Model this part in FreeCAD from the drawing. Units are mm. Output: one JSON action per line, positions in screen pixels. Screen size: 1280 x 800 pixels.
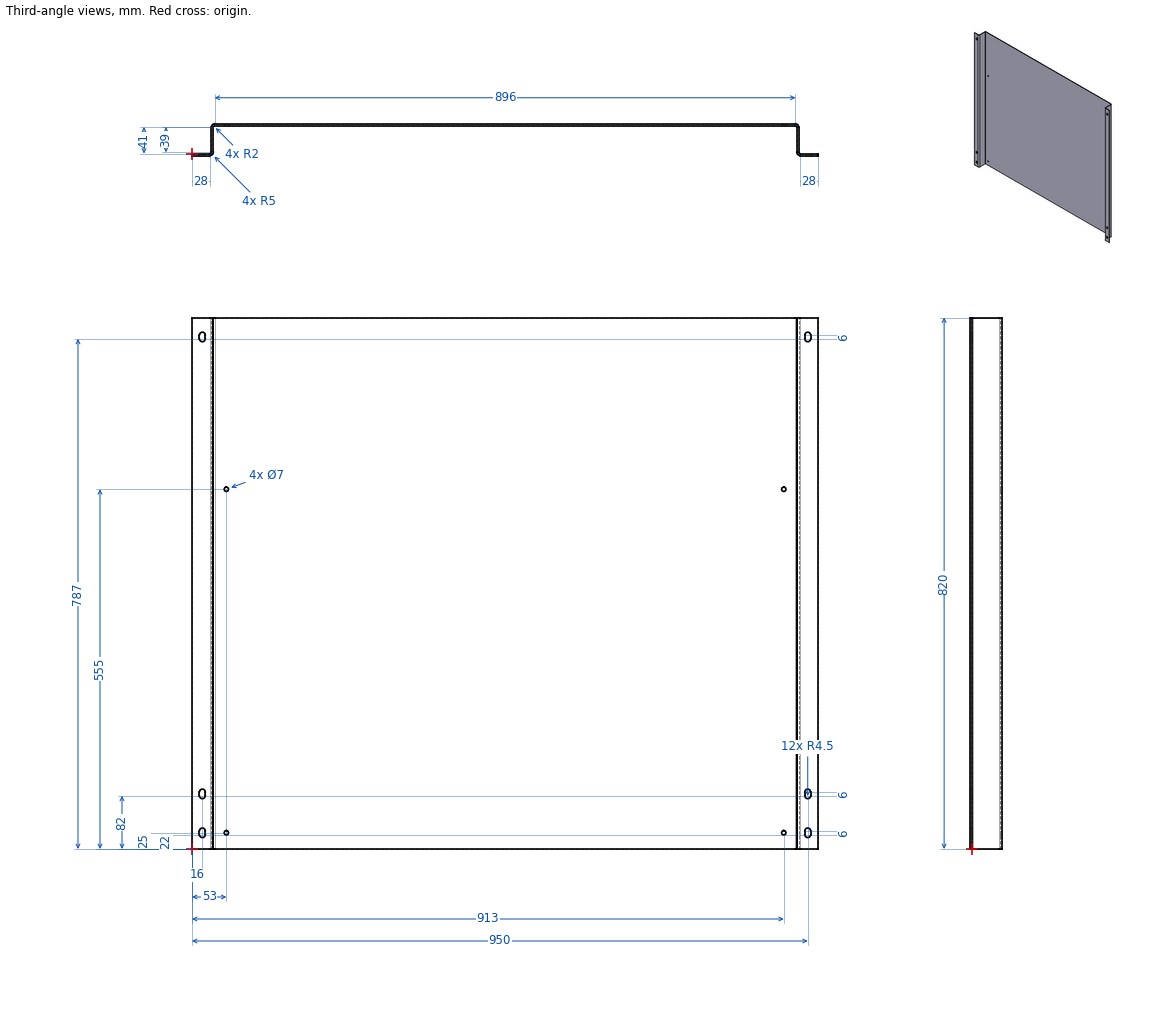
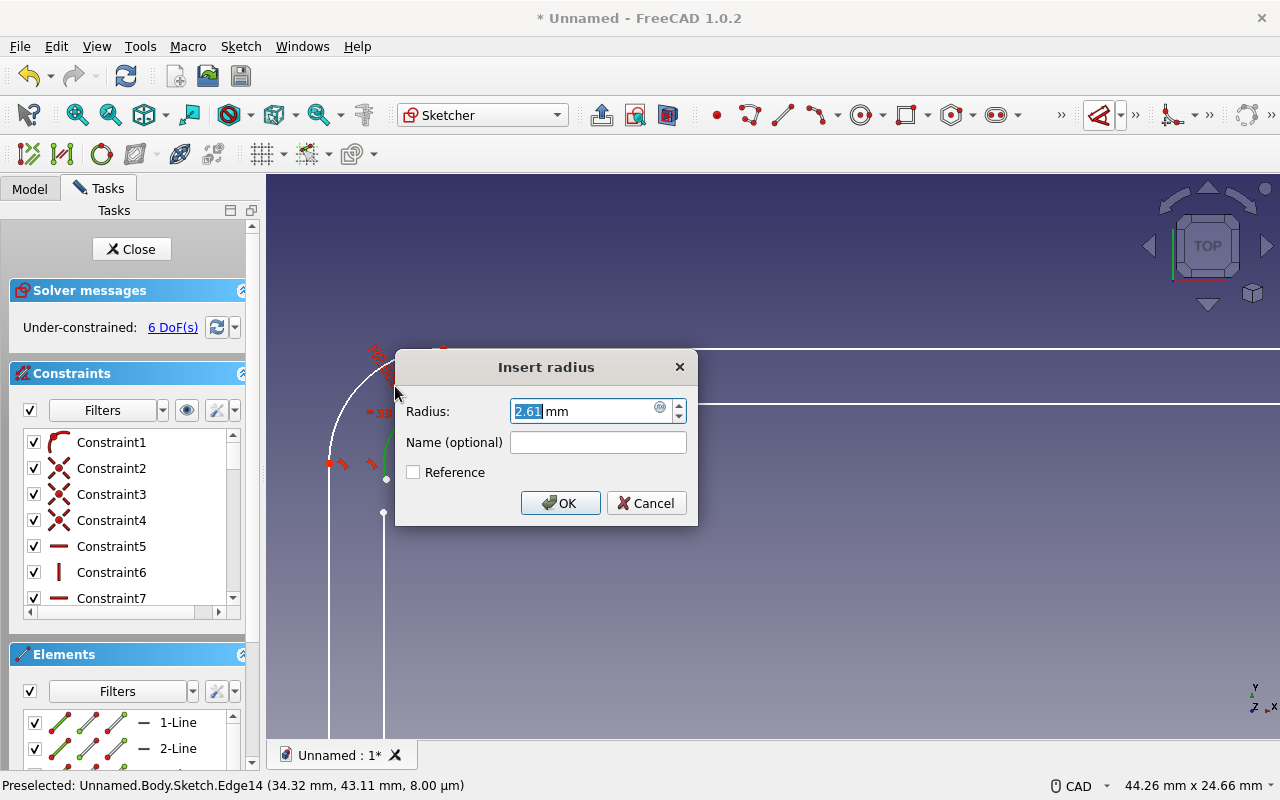
{"action": "type", "text": "2"}
{"action": "key", "text": "Return"}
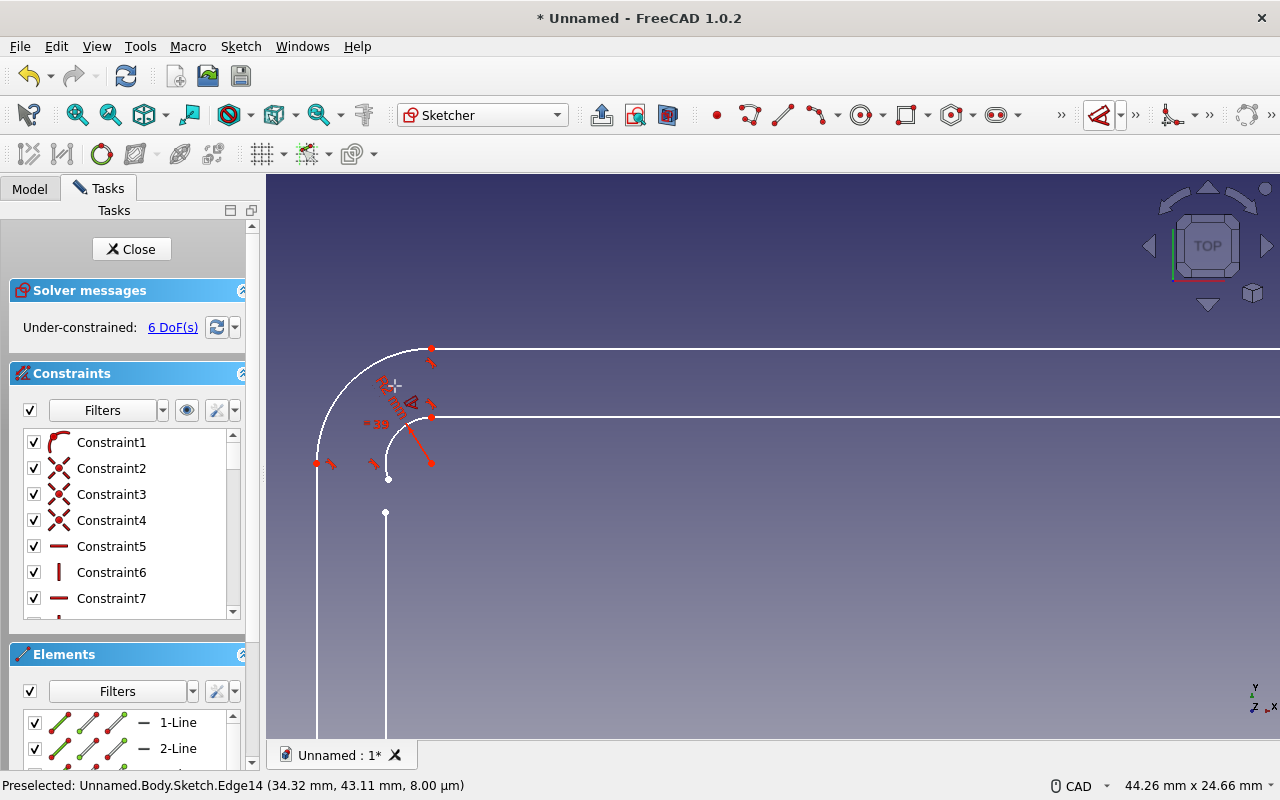
{"action": "scroll", "coordinate": [360, 441], "scroll_direction": "down", "scroll_amount": 17}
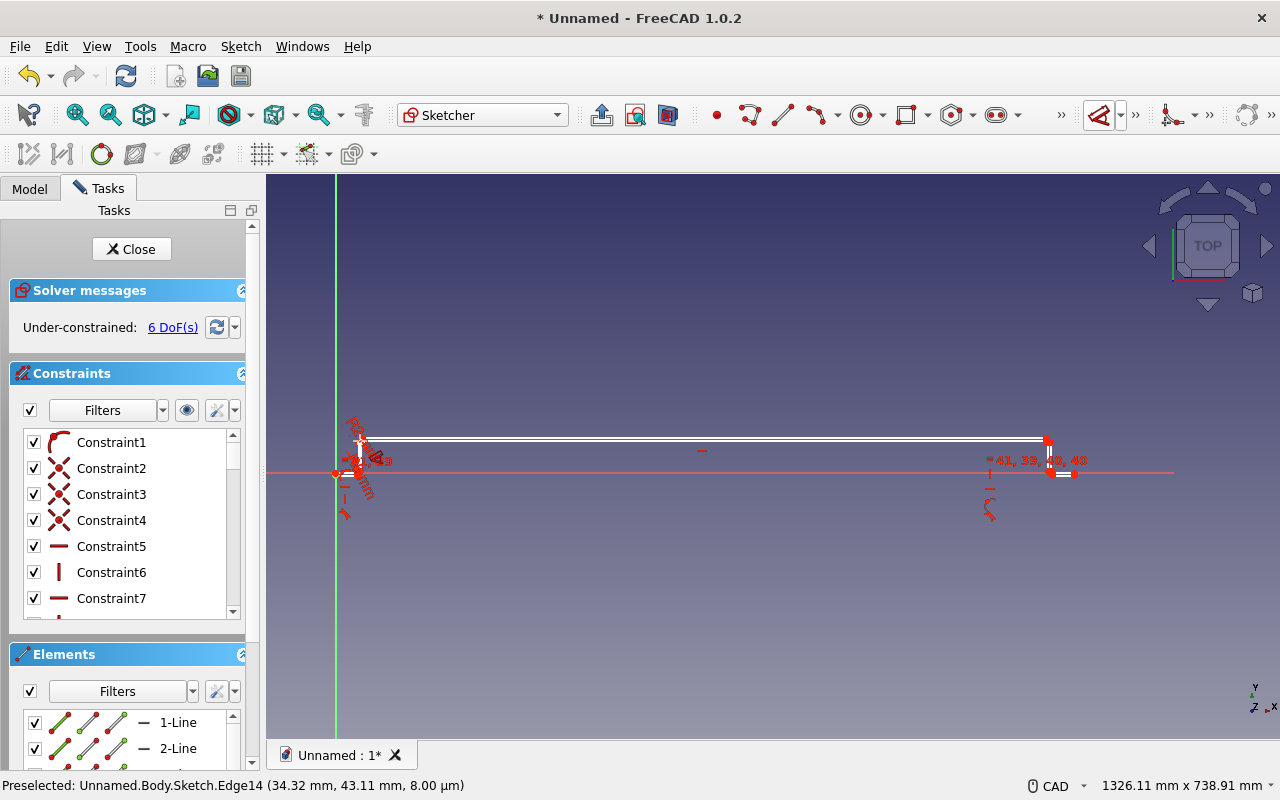
{"action": "scroll", "coordinate": [351, 473], "scroll_direction": "up", "scroll_amount": 9}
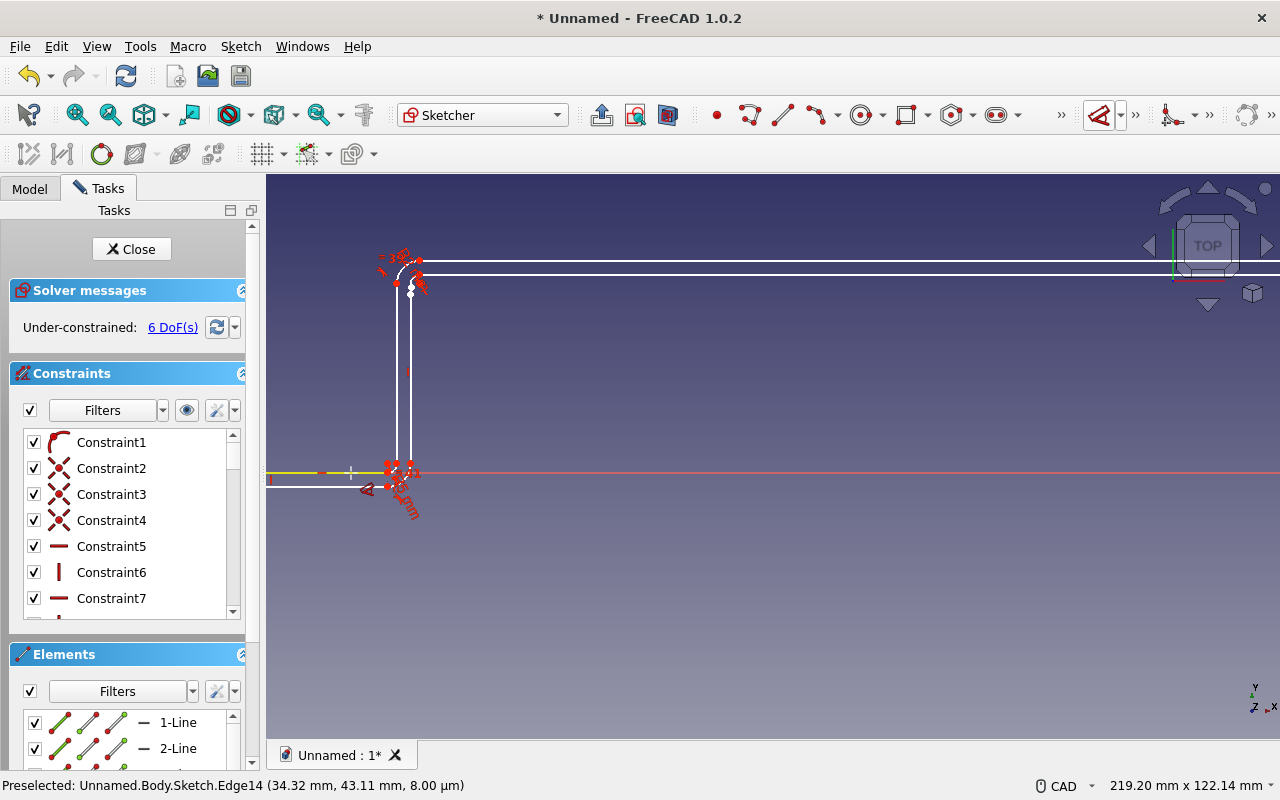
{"action": "left_click", "coordinate": [349, 473]}
{"action": "left_click", "coordinate": [319, 507]}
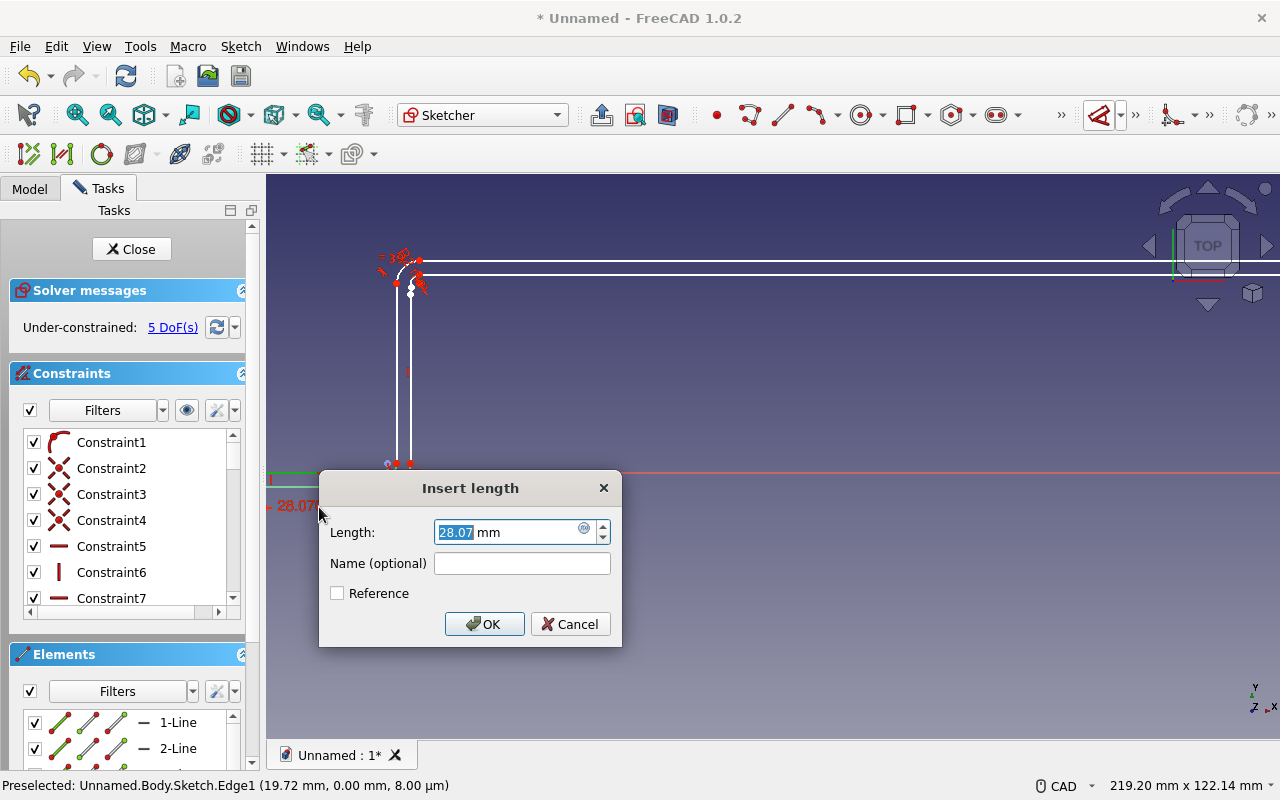
{"action": "type", "text": "28"}
{"action": "key", "text": "Return"}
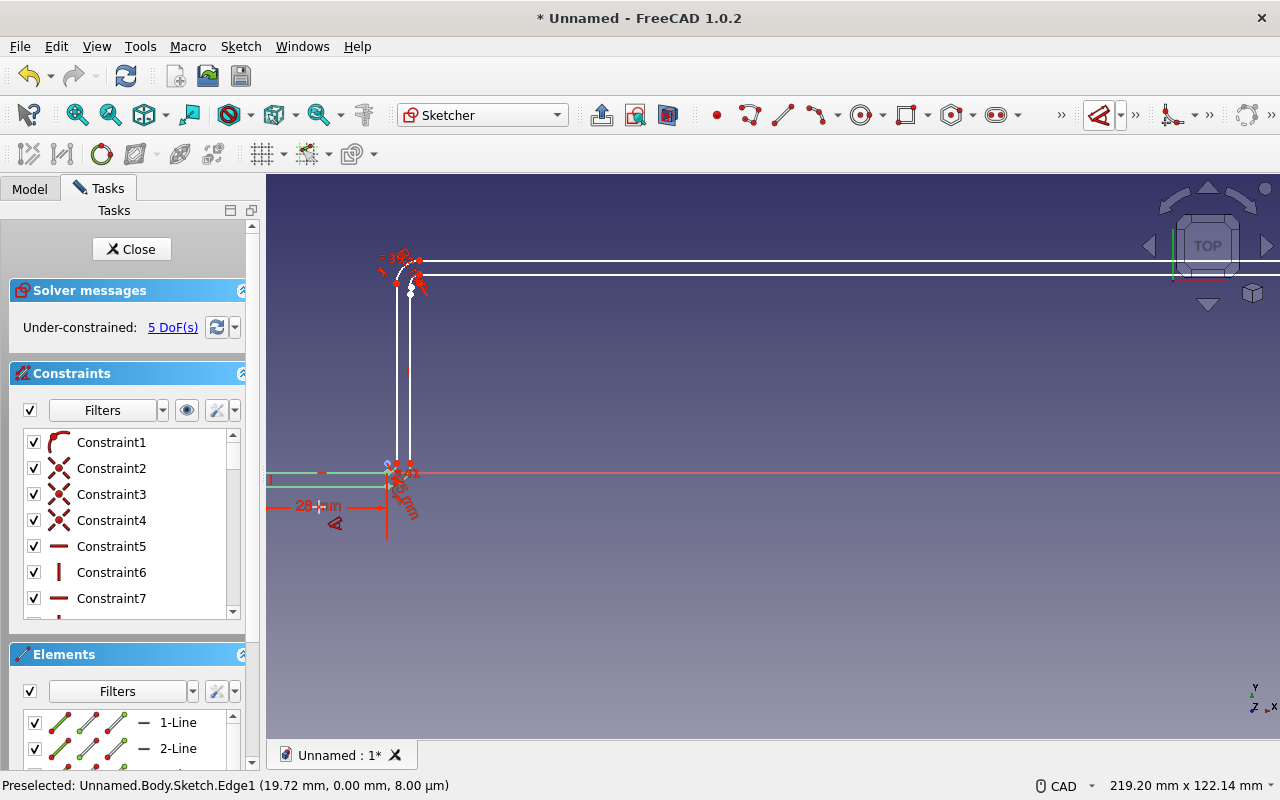
{"action": "left_click", "coordinate": [410, 413]}
{"action": "left_click", "coordinate": [376, 379]}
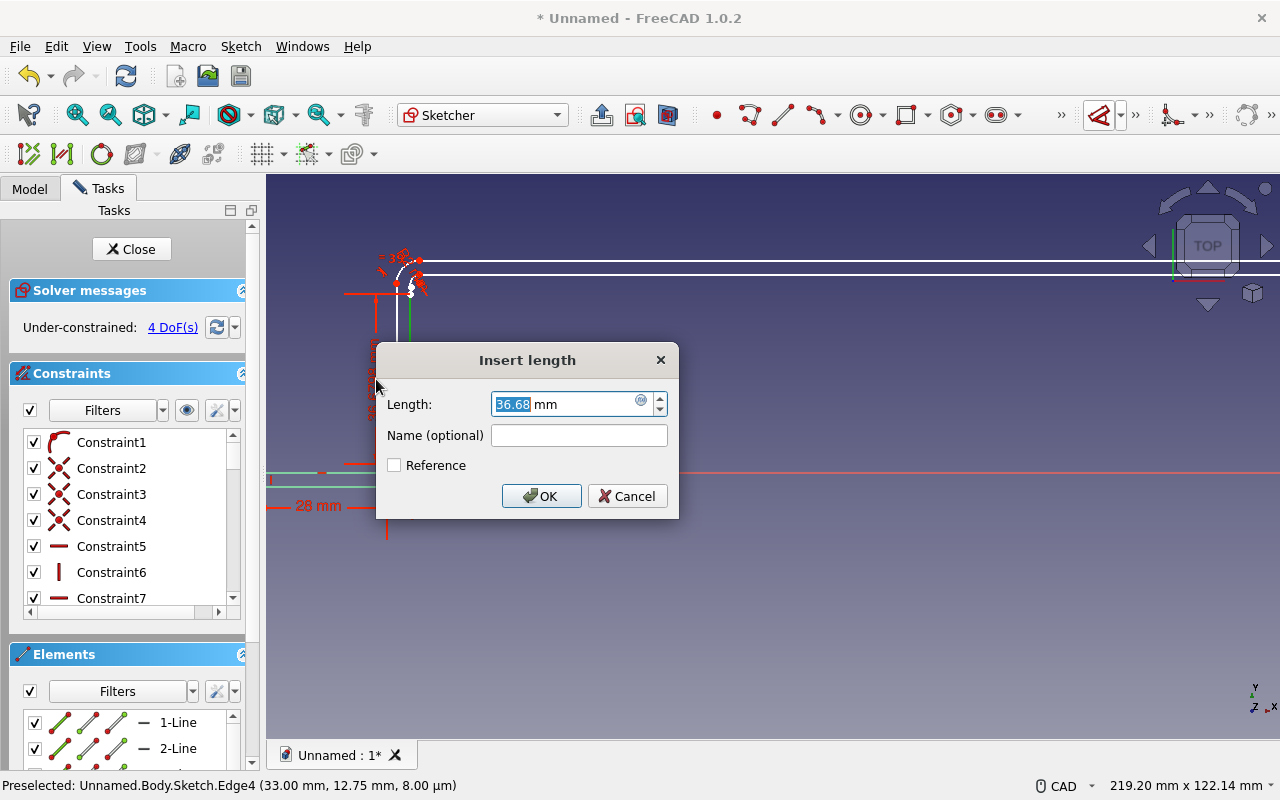
{"action": "type", "text": "39"}
{"action": "key", "text": "Return"}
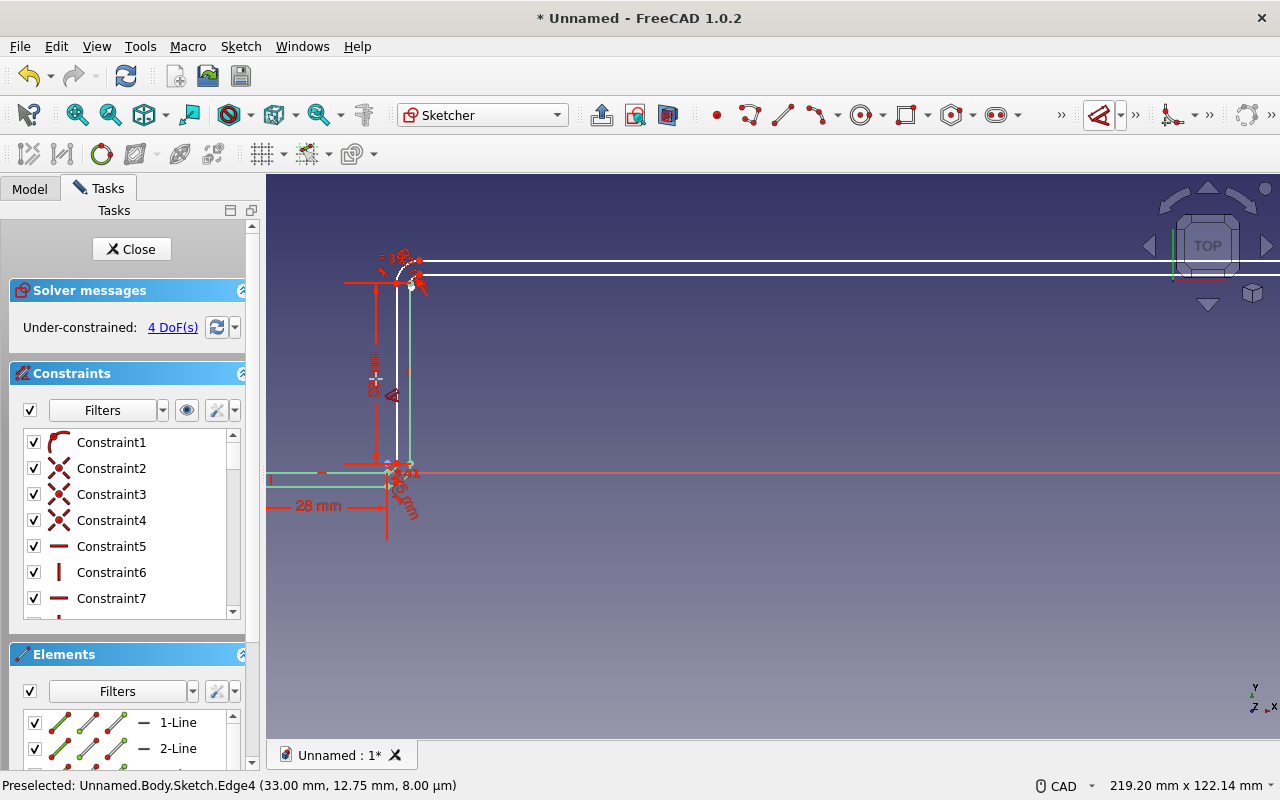
{"action": "scroll", "coordinate": [425, 469], "scroll_direction": "down", "scroll_amount": 10}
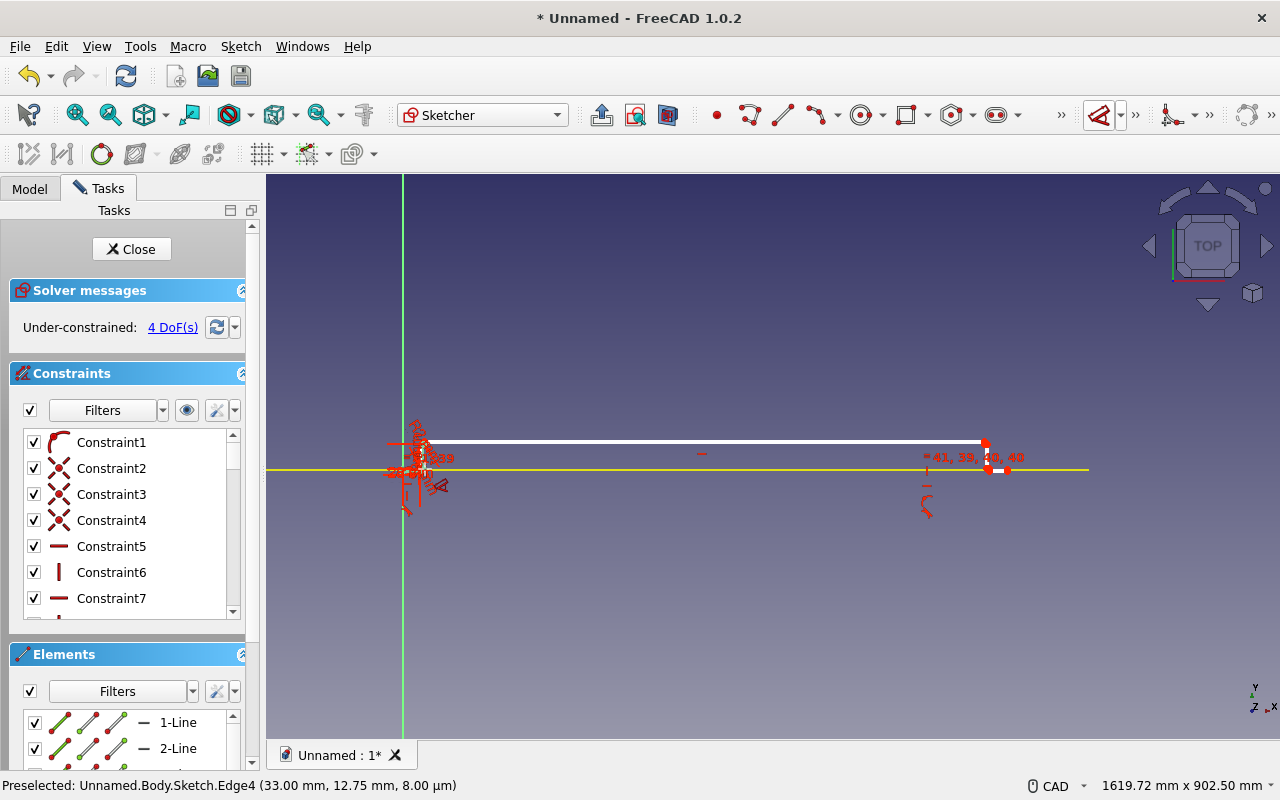
{"action": "scroll", "coordinate": [986, 452], "scroll_direction": "up", "scroll_amount": 10}